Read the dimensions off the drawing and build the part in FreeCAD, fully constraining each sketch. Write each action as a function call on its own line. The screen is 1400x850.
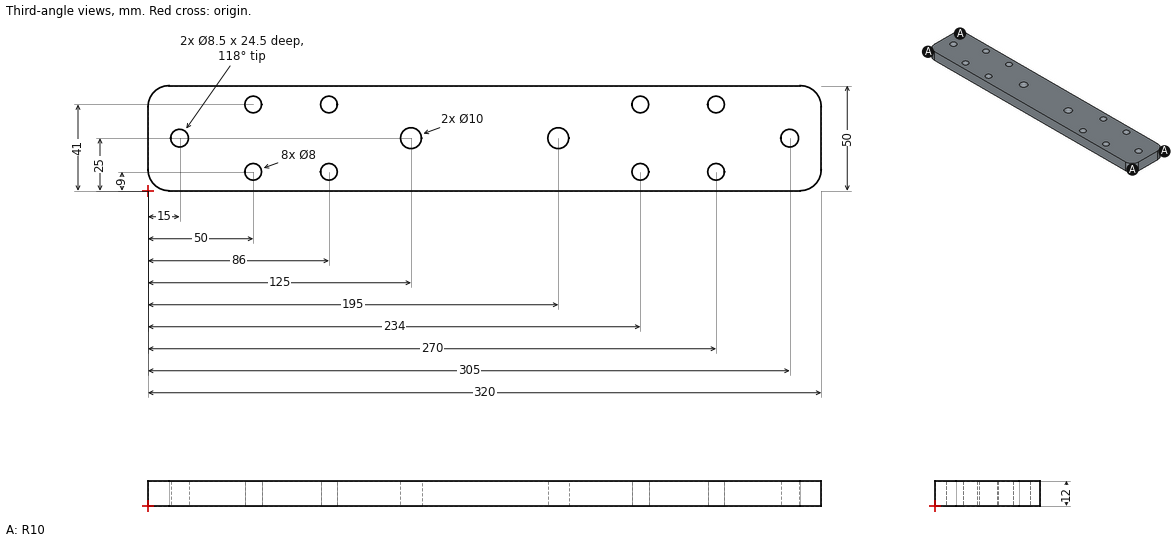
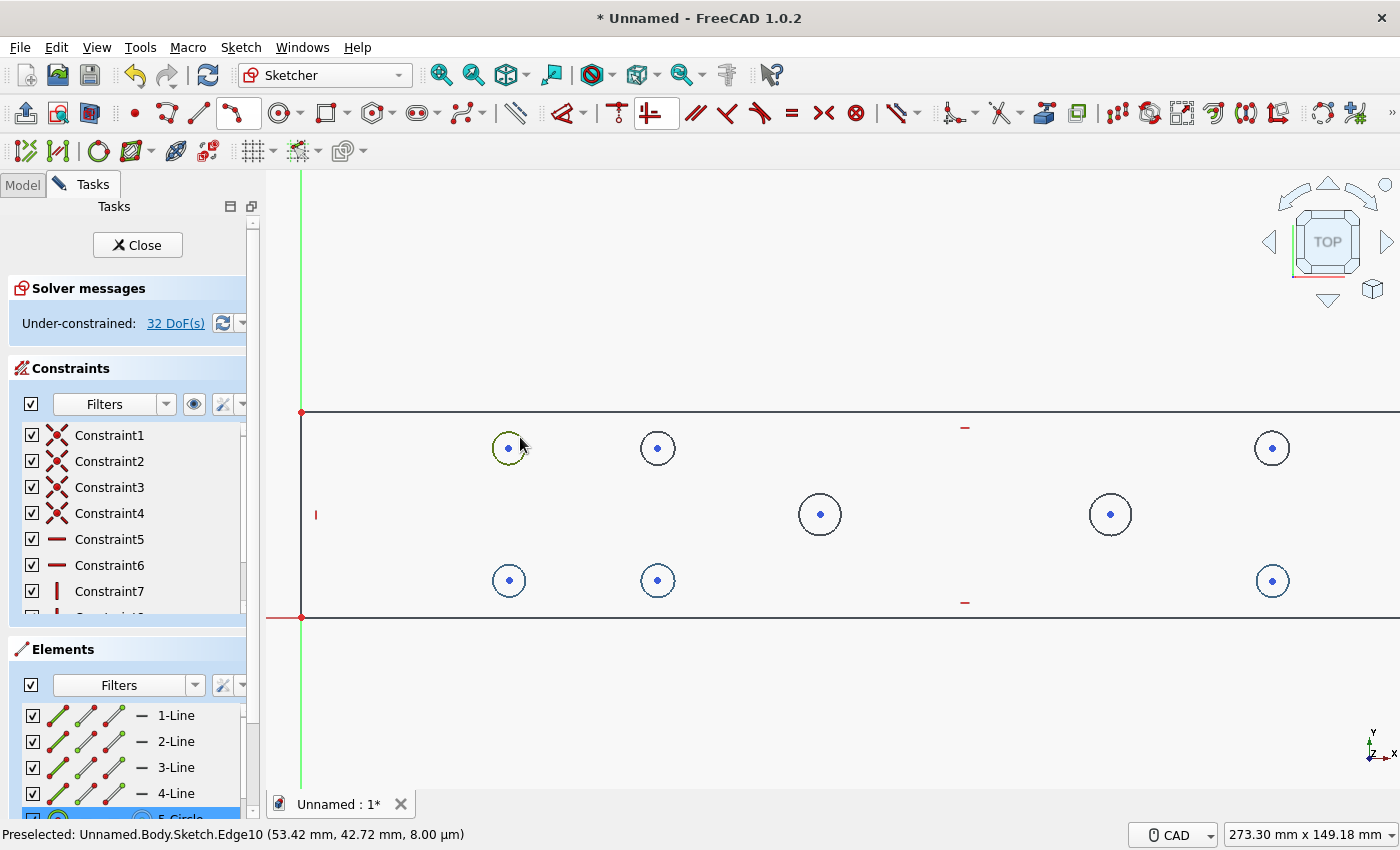
click(670, 436)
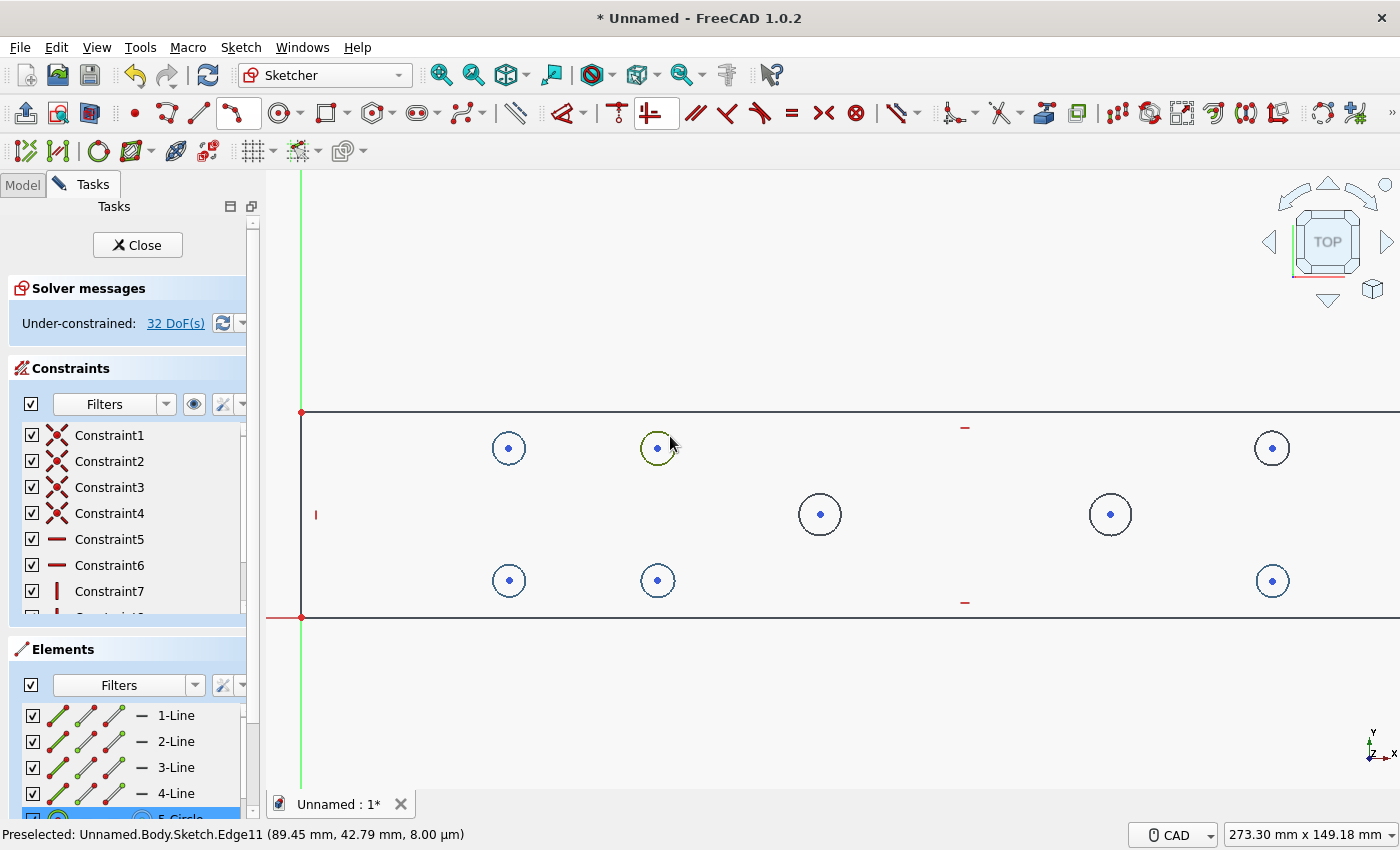
scroll(520, 437, down, 3)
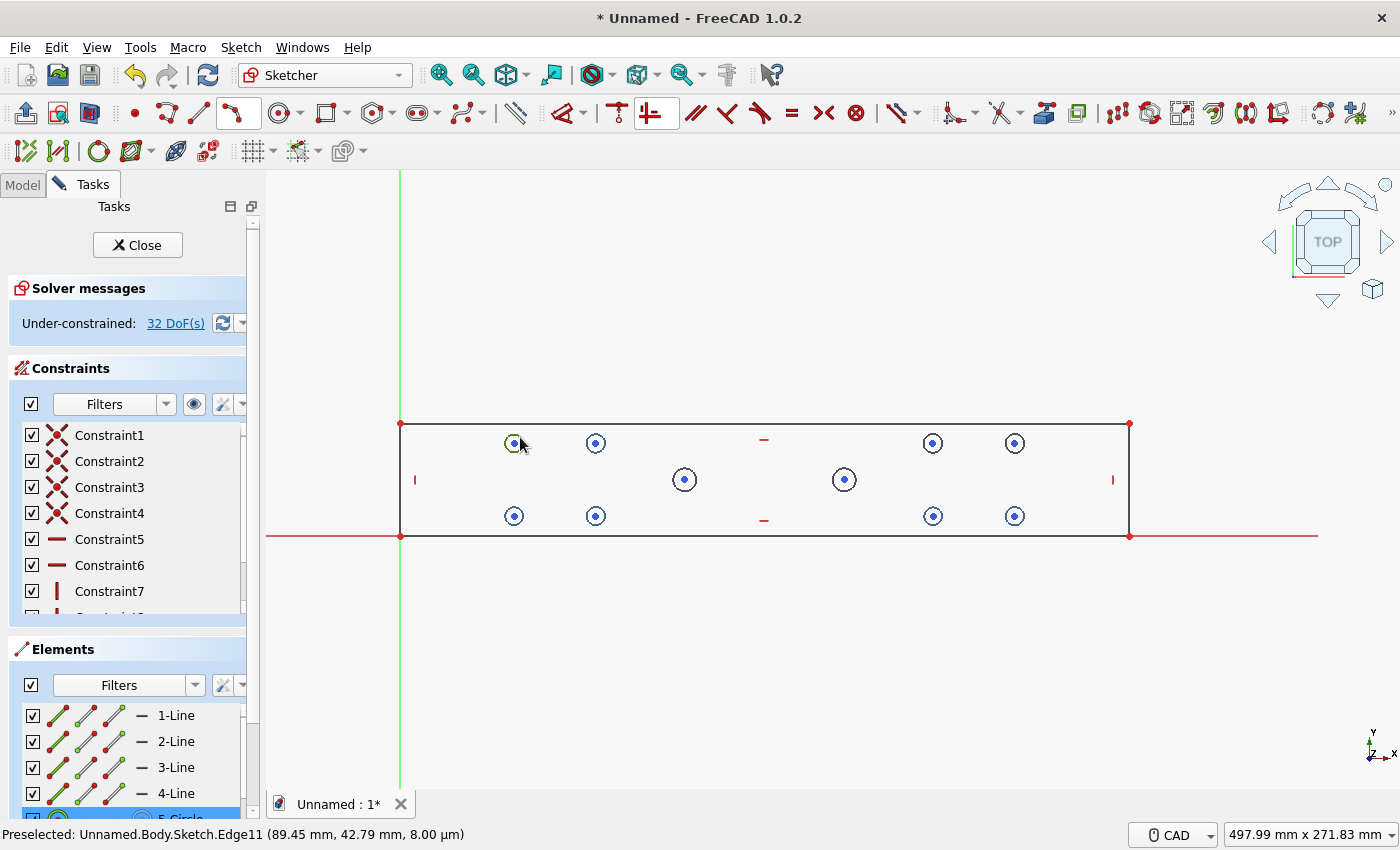
scroll(940, 437, up, 2)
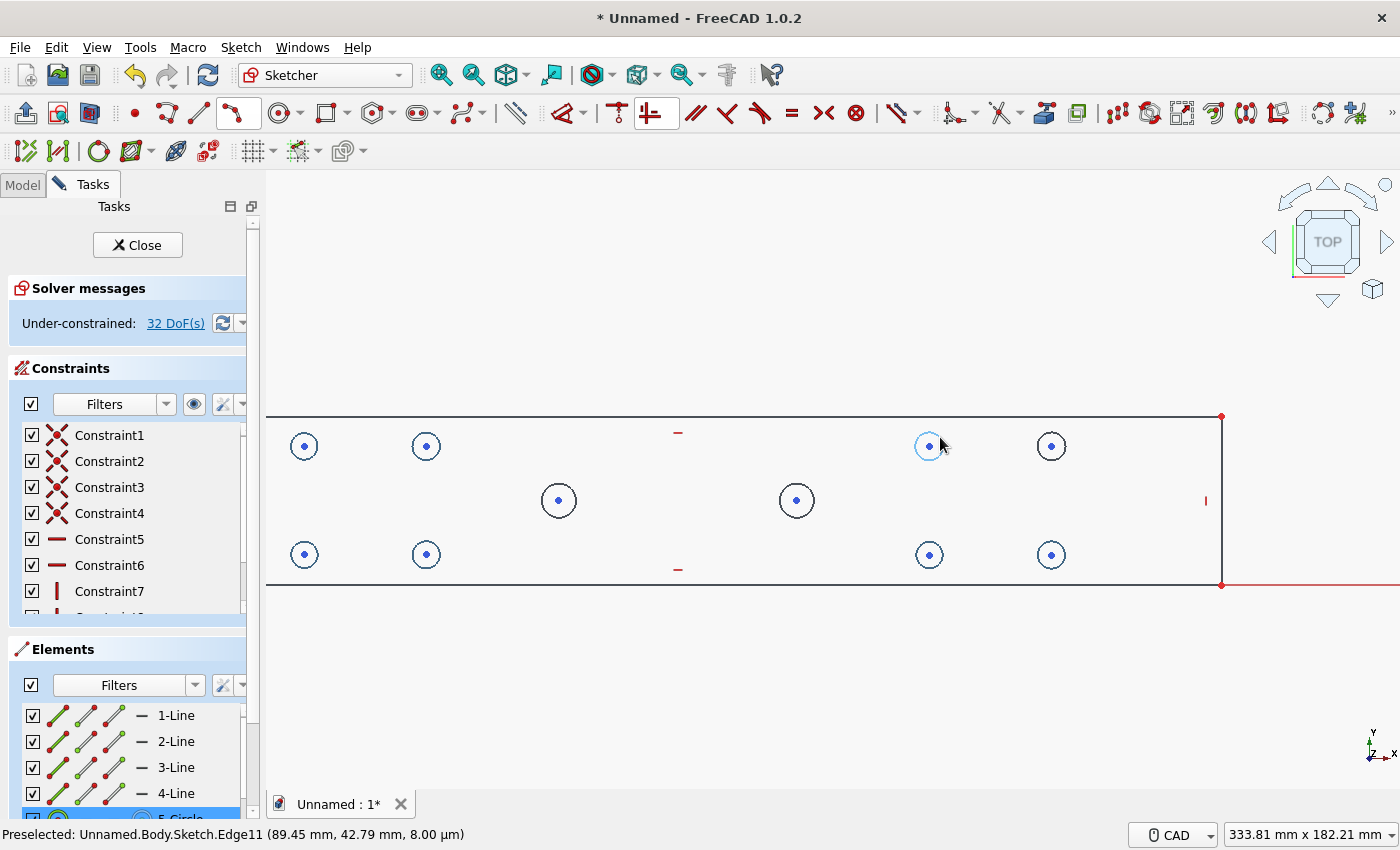
click(939, 437)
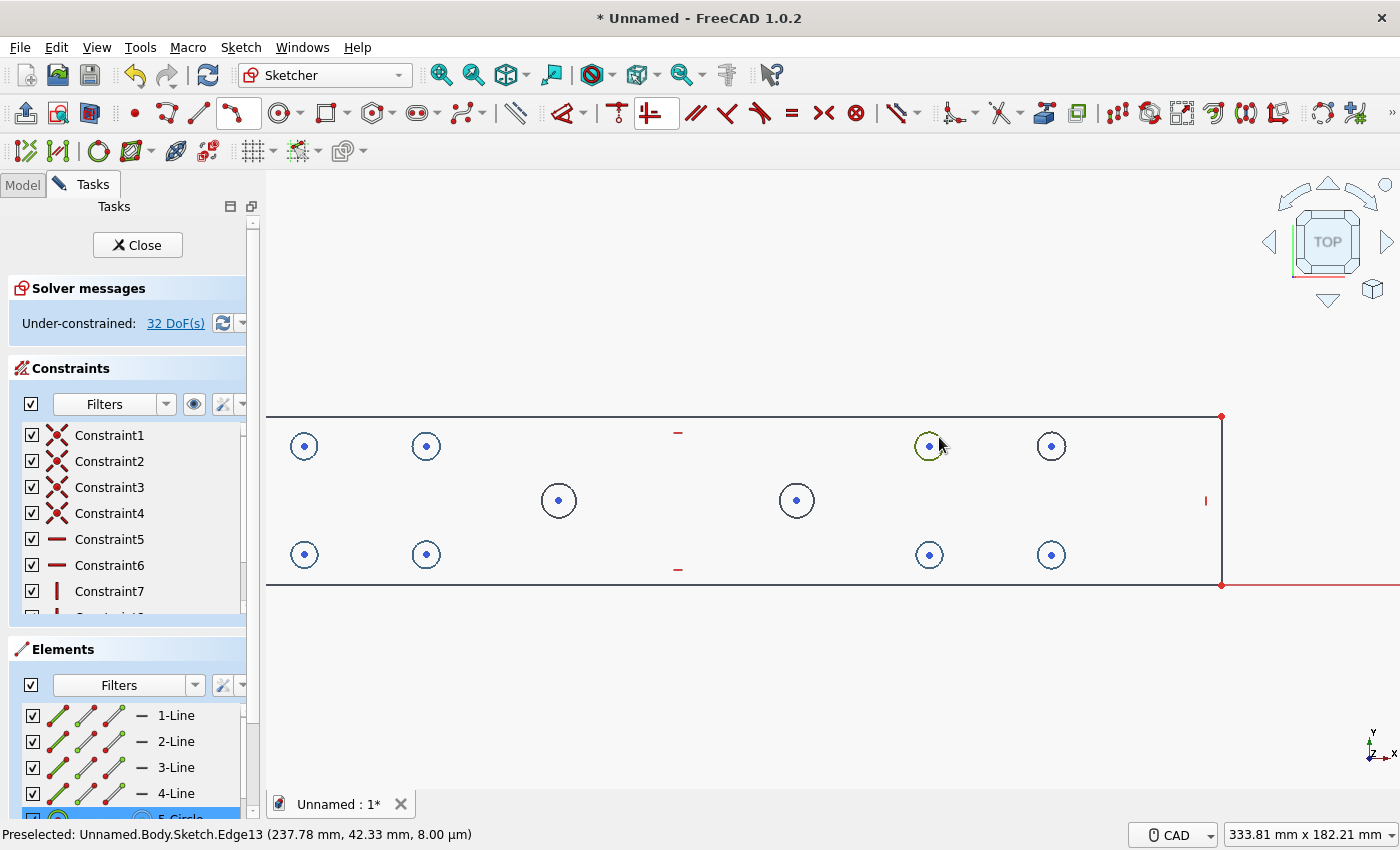
click(1061, 437)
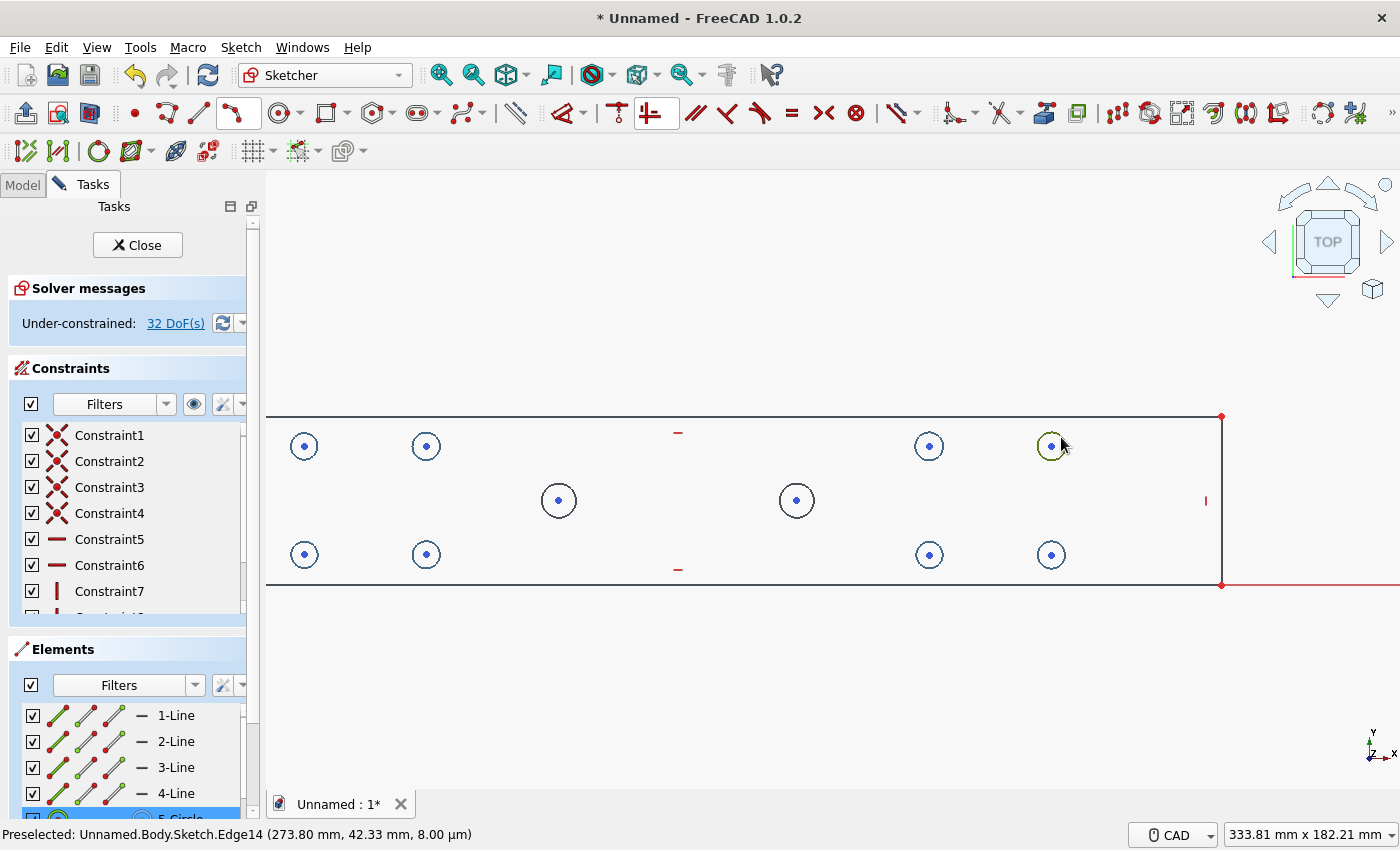
click(792, 114)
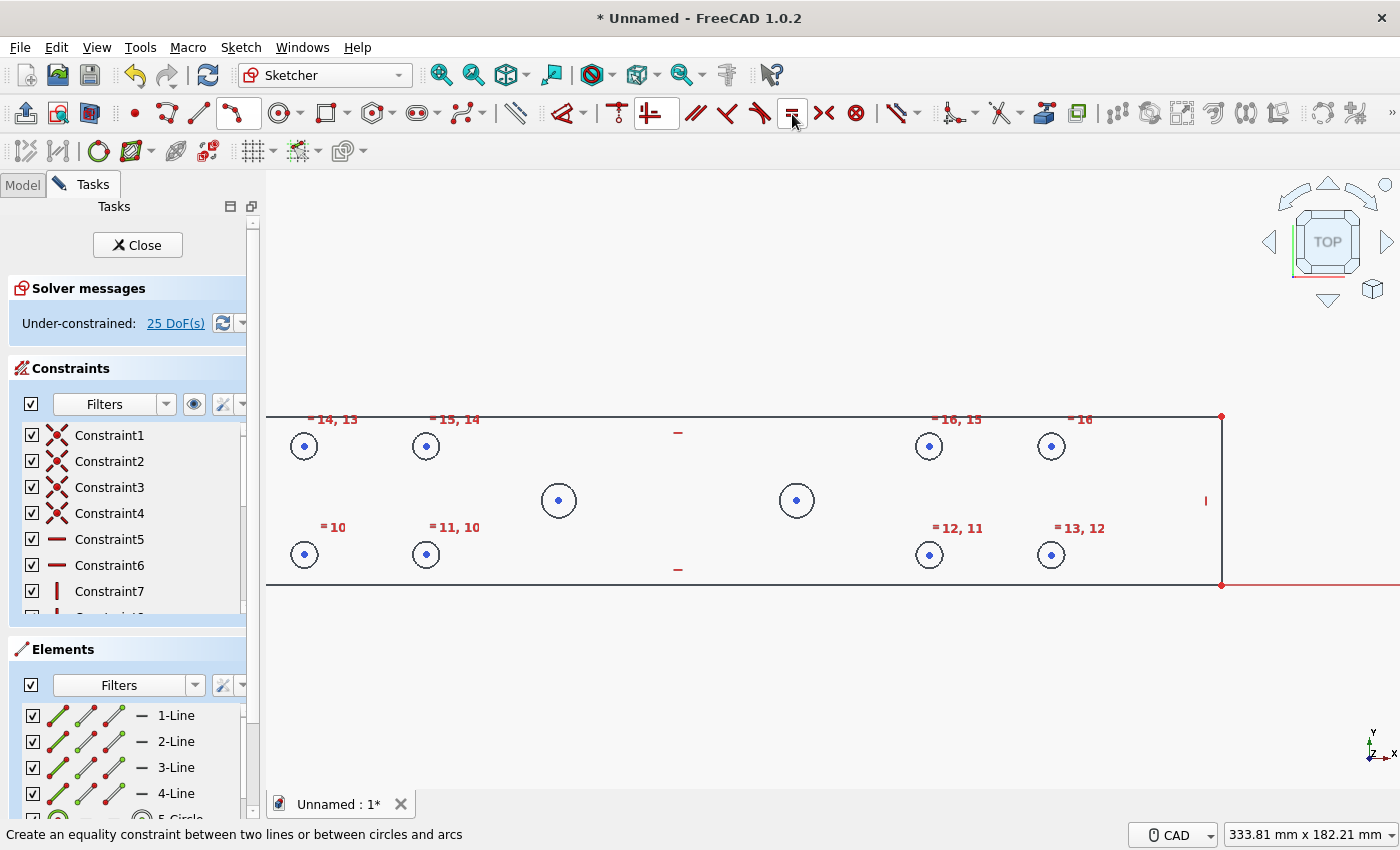
click(571, 489)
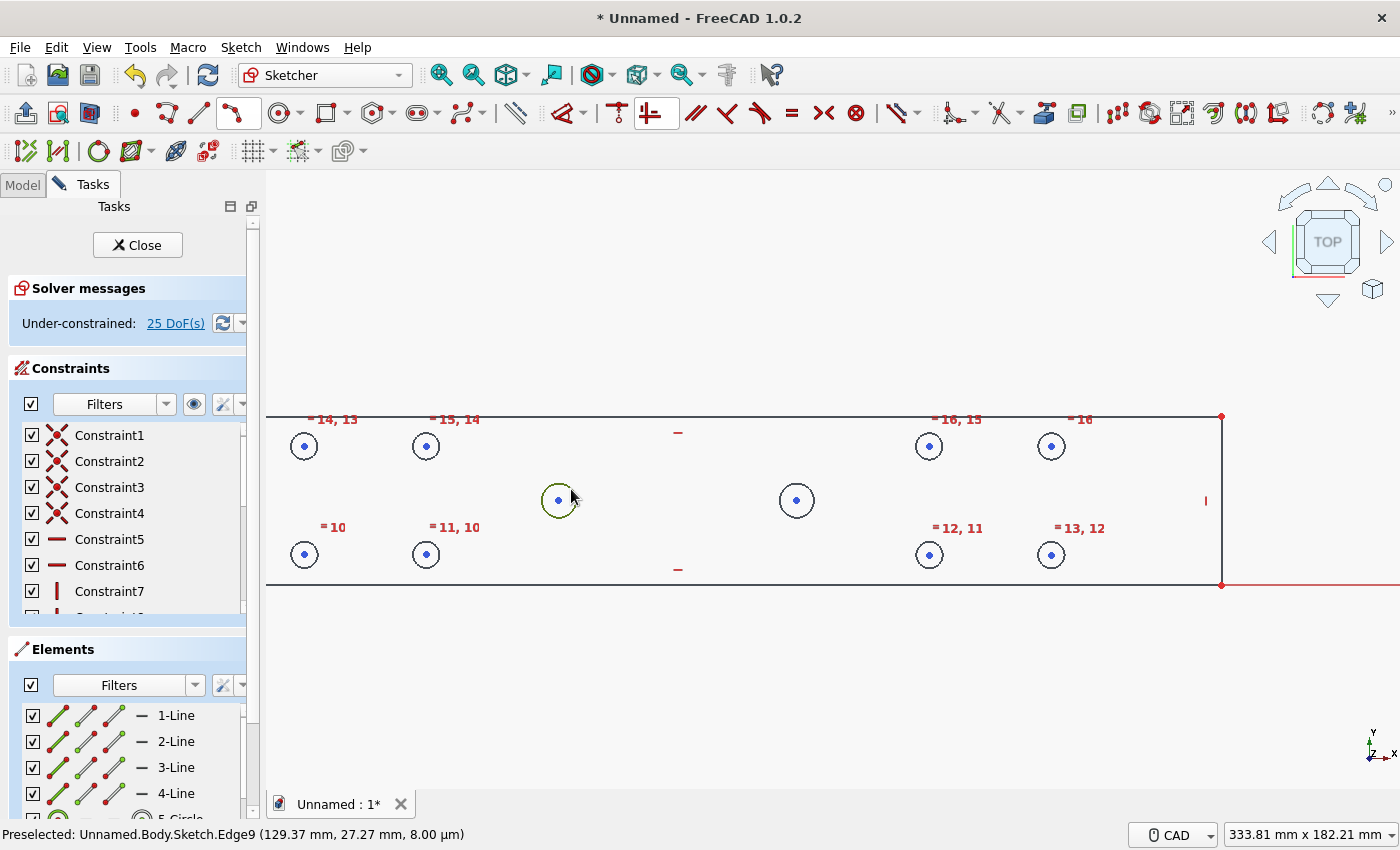
click(809, 489)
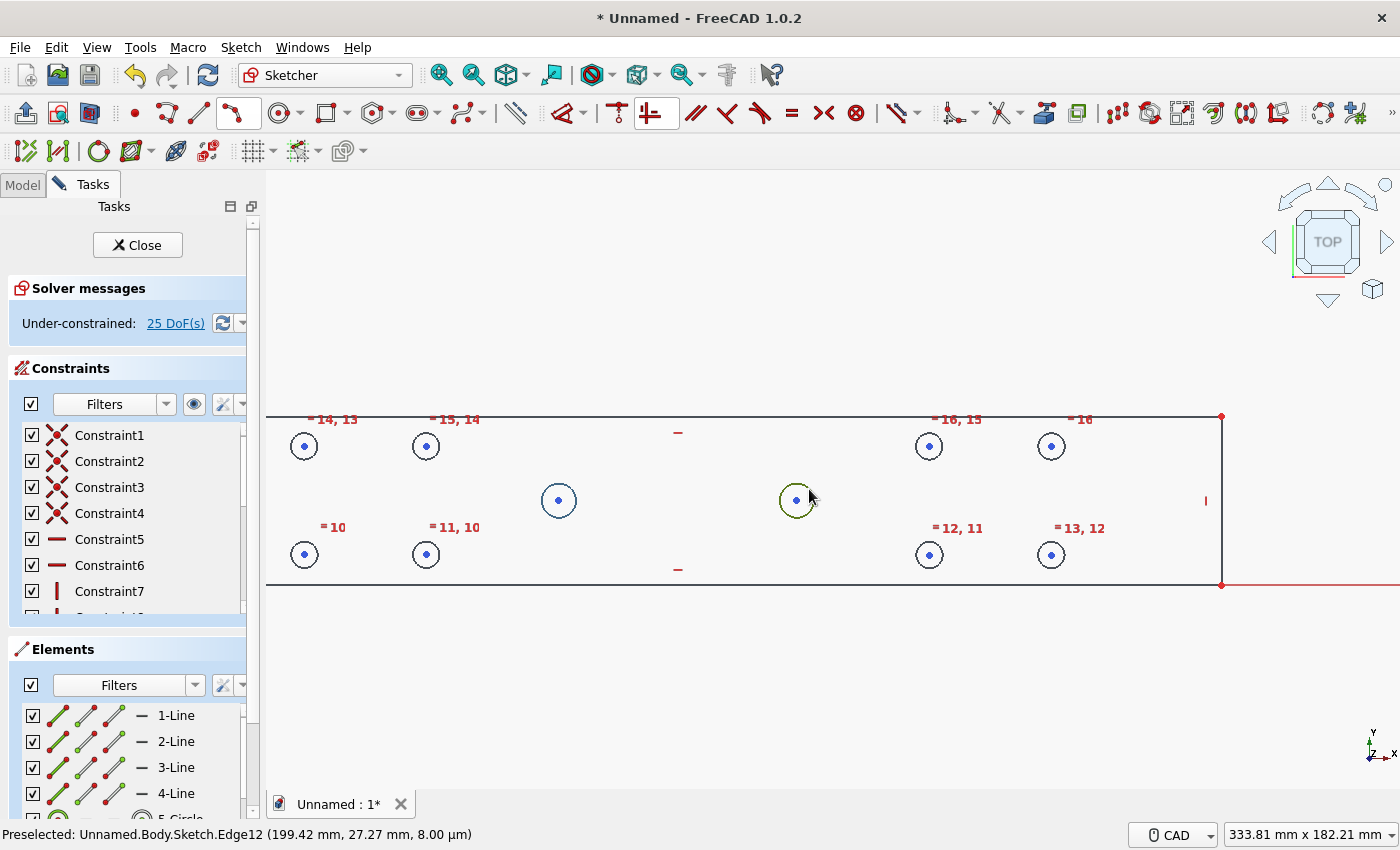
key(e)